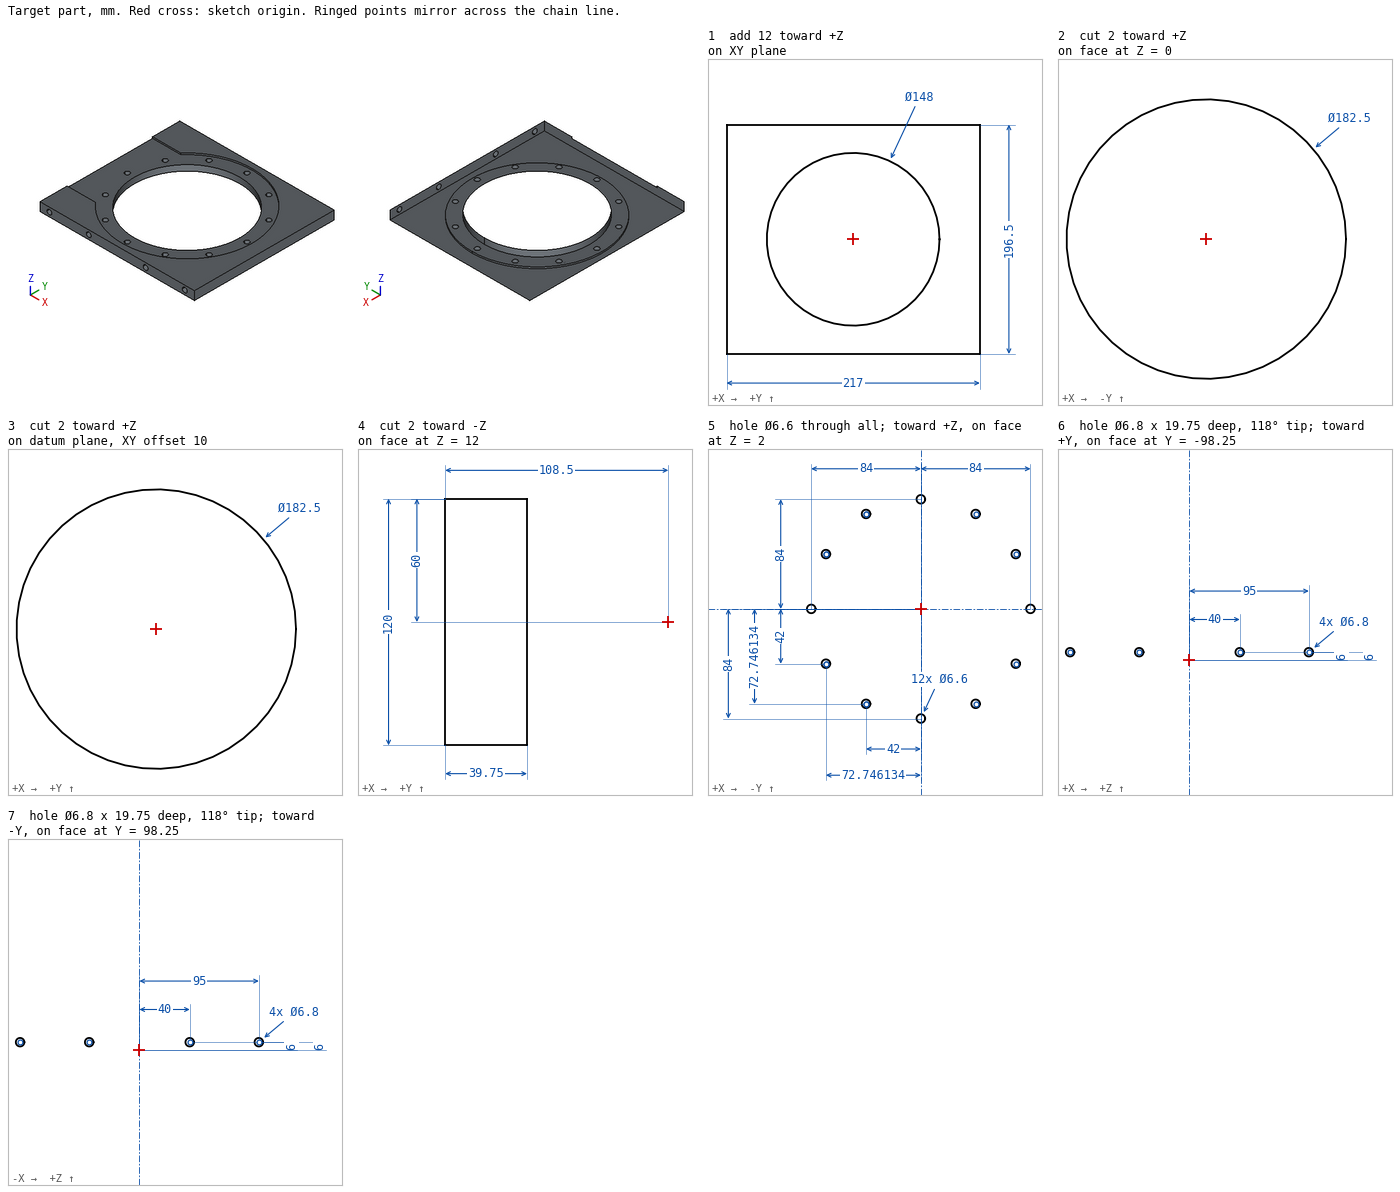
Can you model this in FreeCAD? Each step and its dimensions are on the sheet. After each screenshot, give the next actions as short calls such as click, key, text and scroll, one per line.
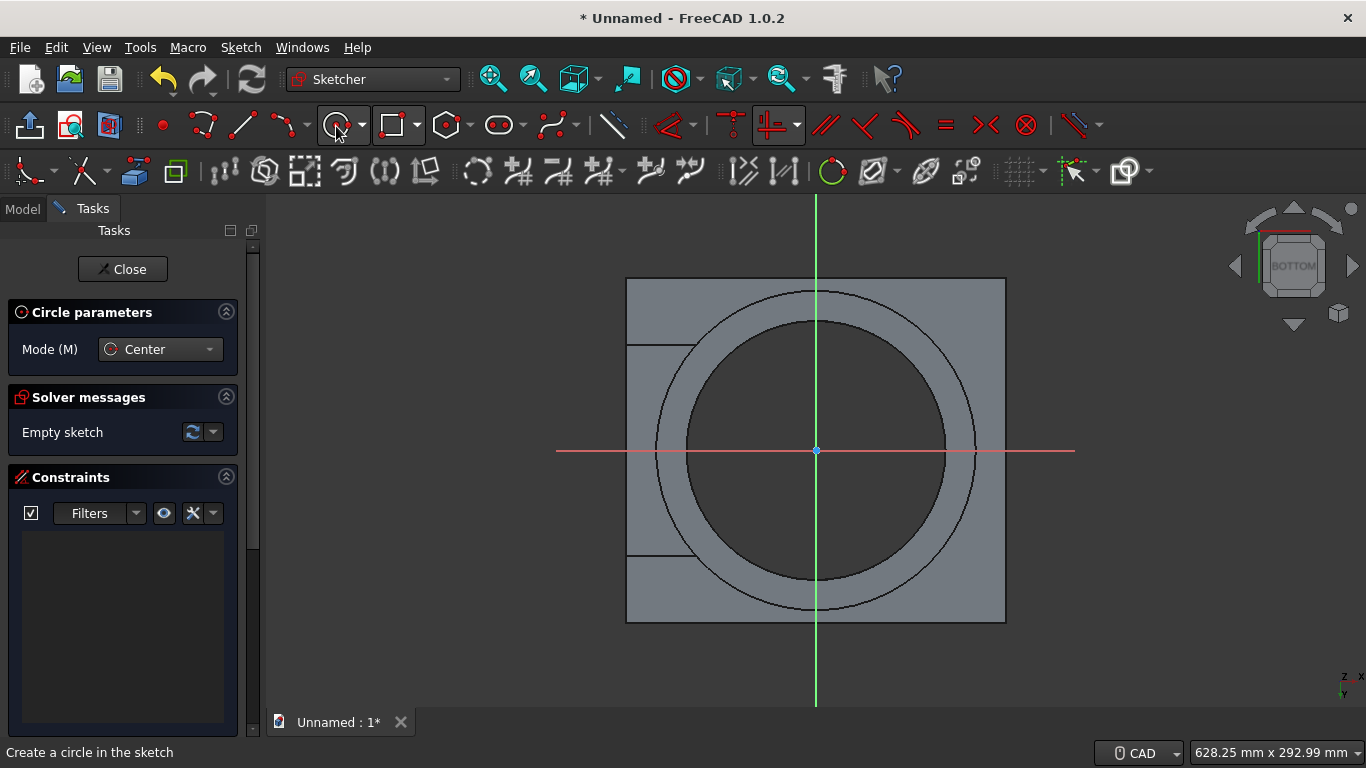
scroll(816, 598, up, 7)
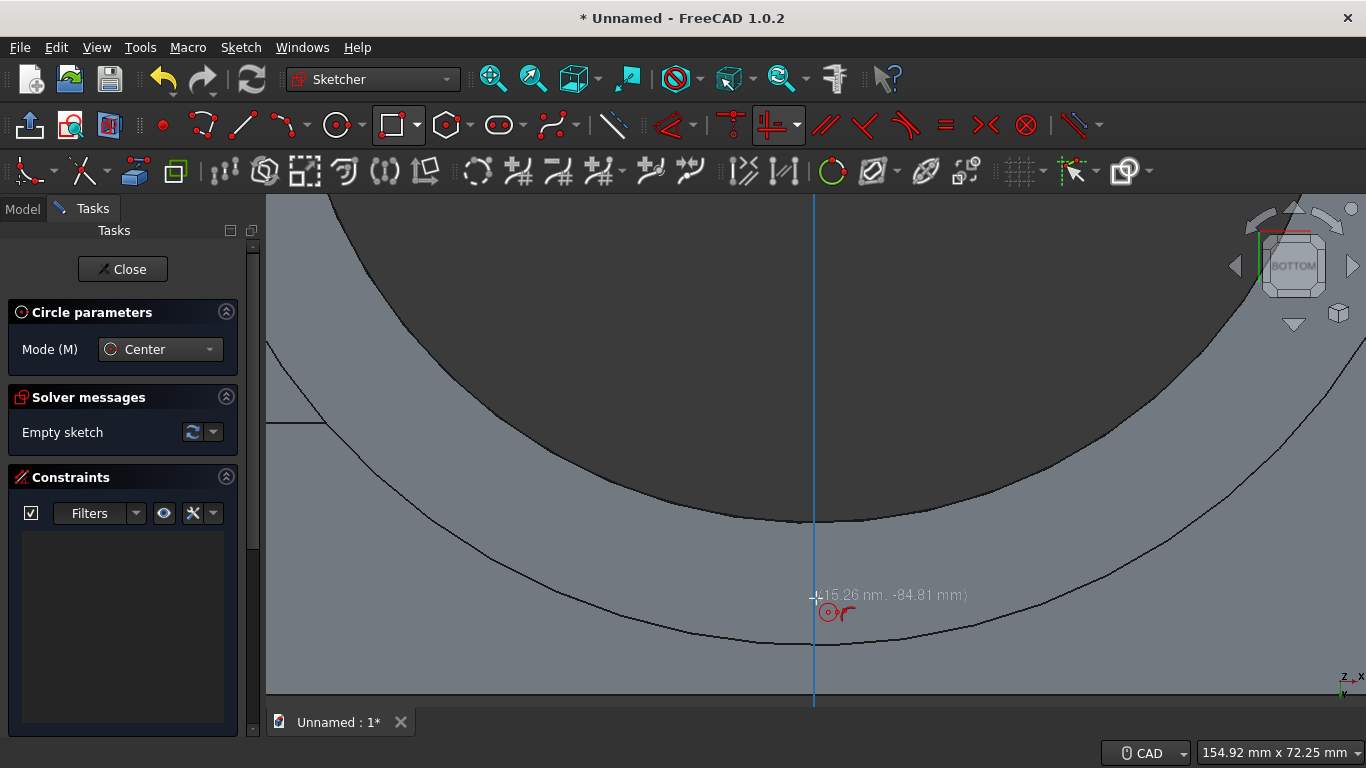
scroll(726, 599, down, 7)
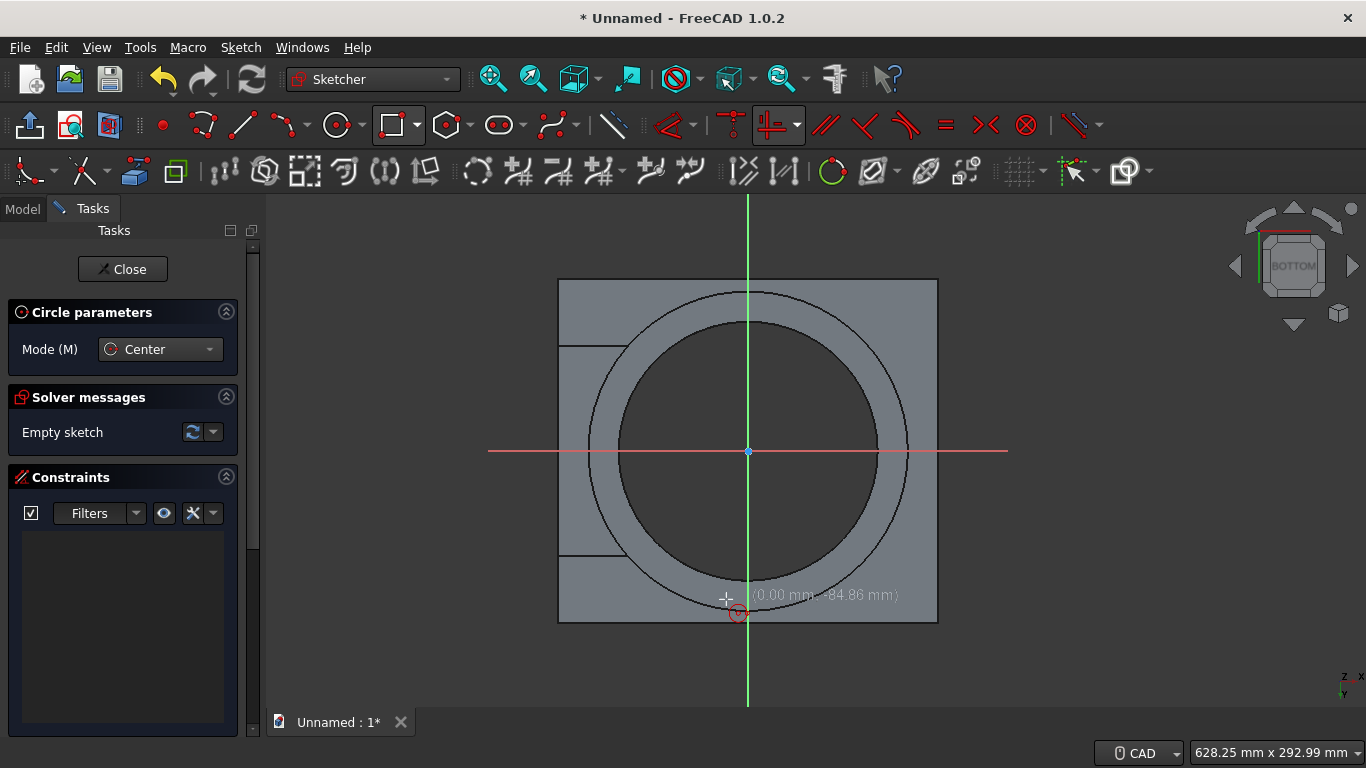
click(748, 598)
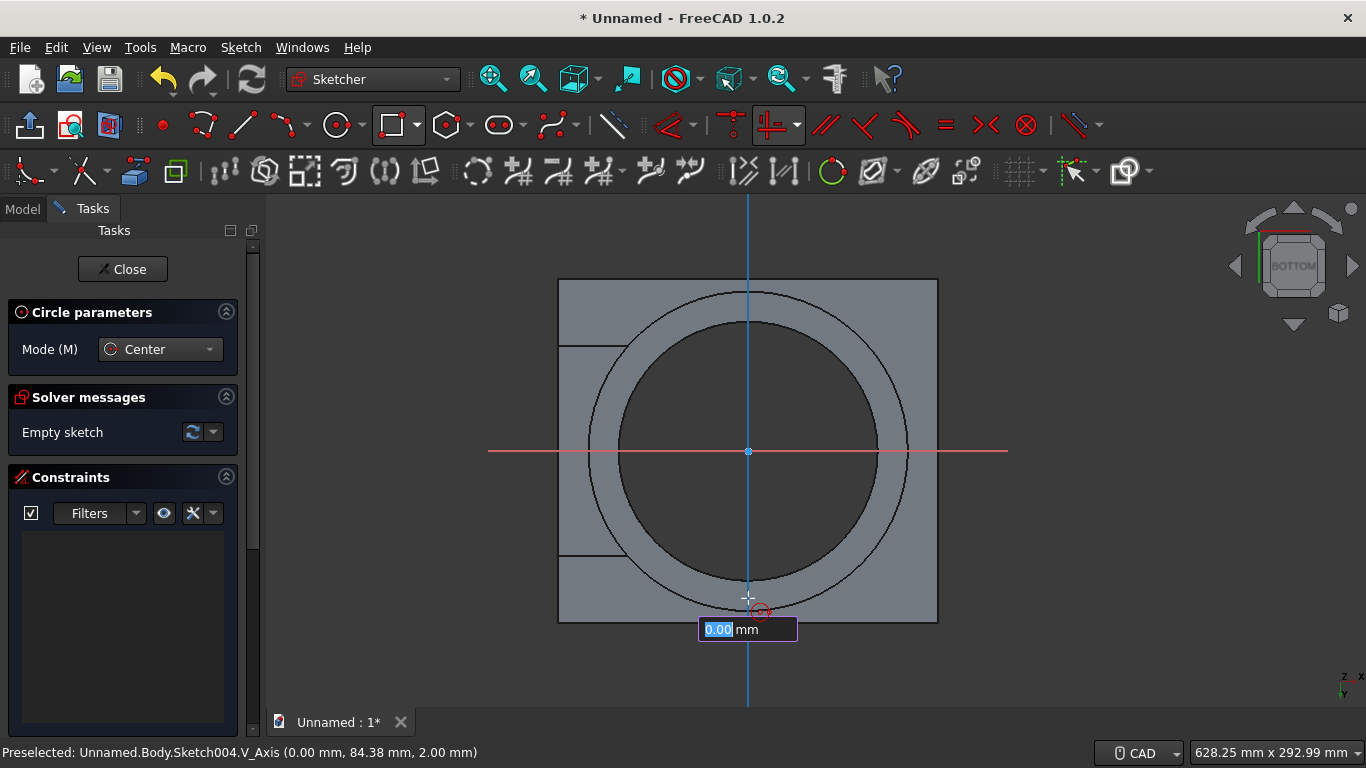
scroll(754, 596, up, 6)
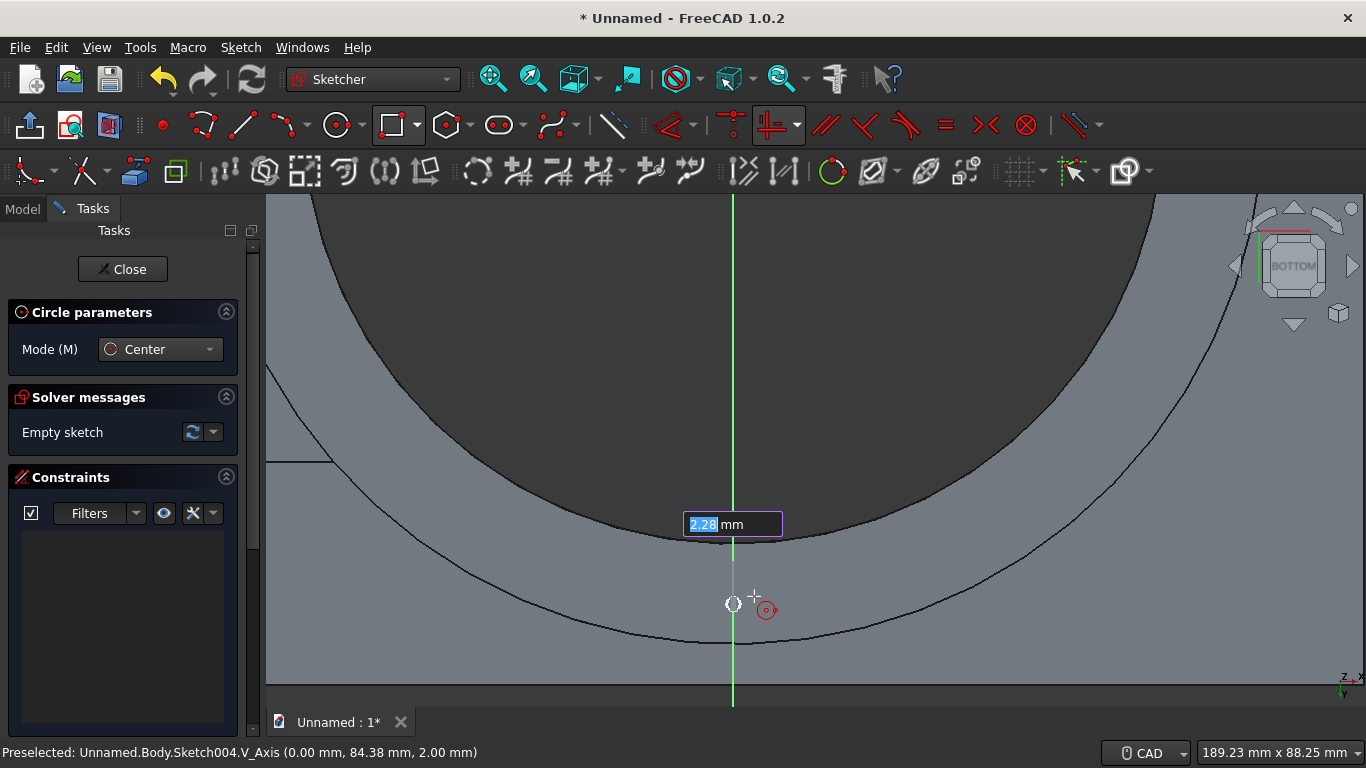
click(752, 595)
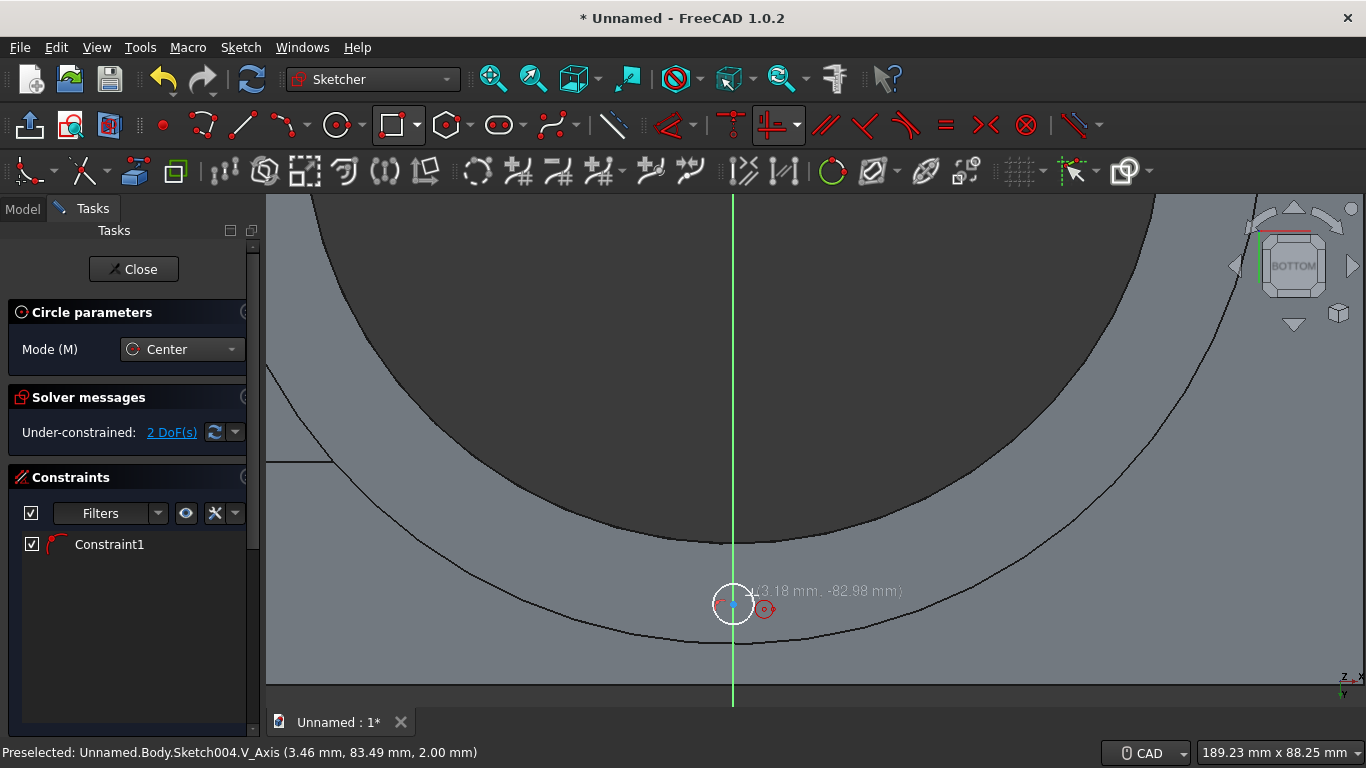
click(489, 536)
click(503, 523)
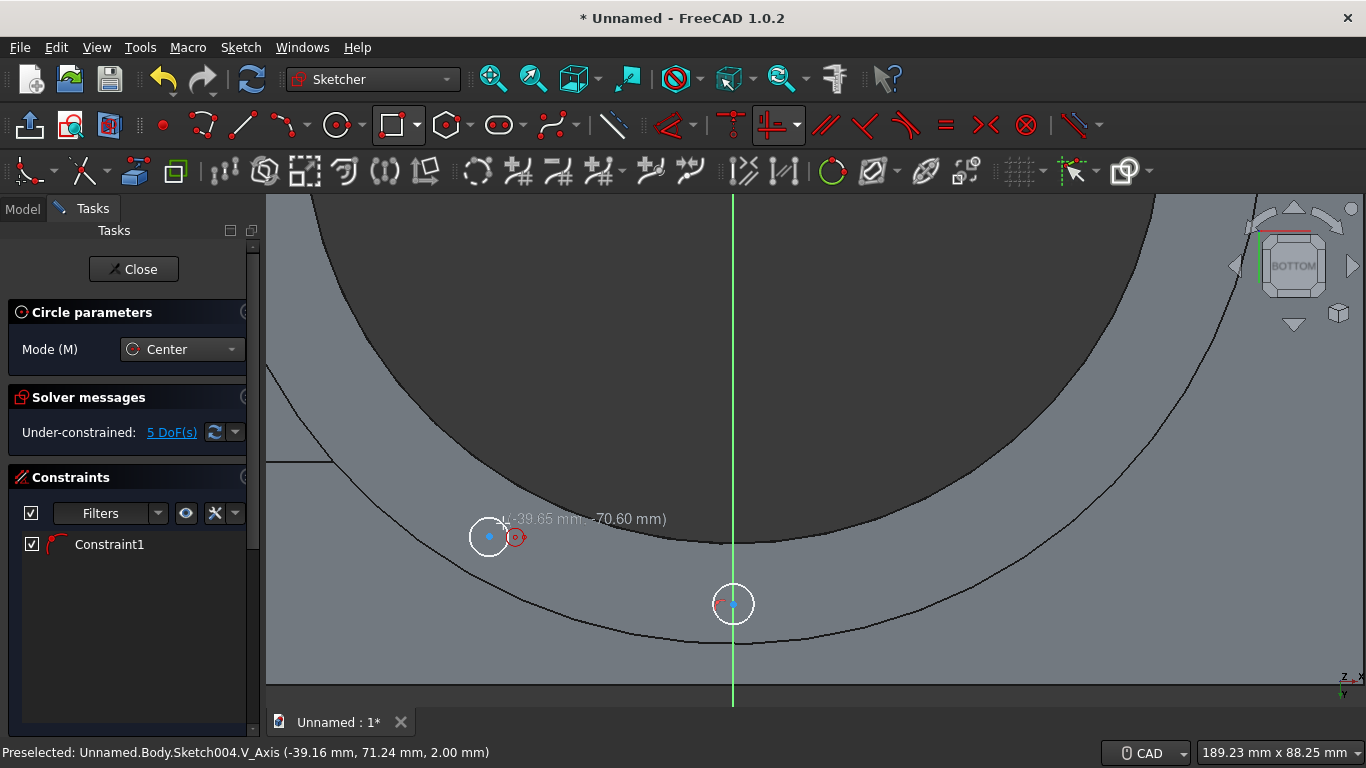
click(311, 358)
click(324, 344)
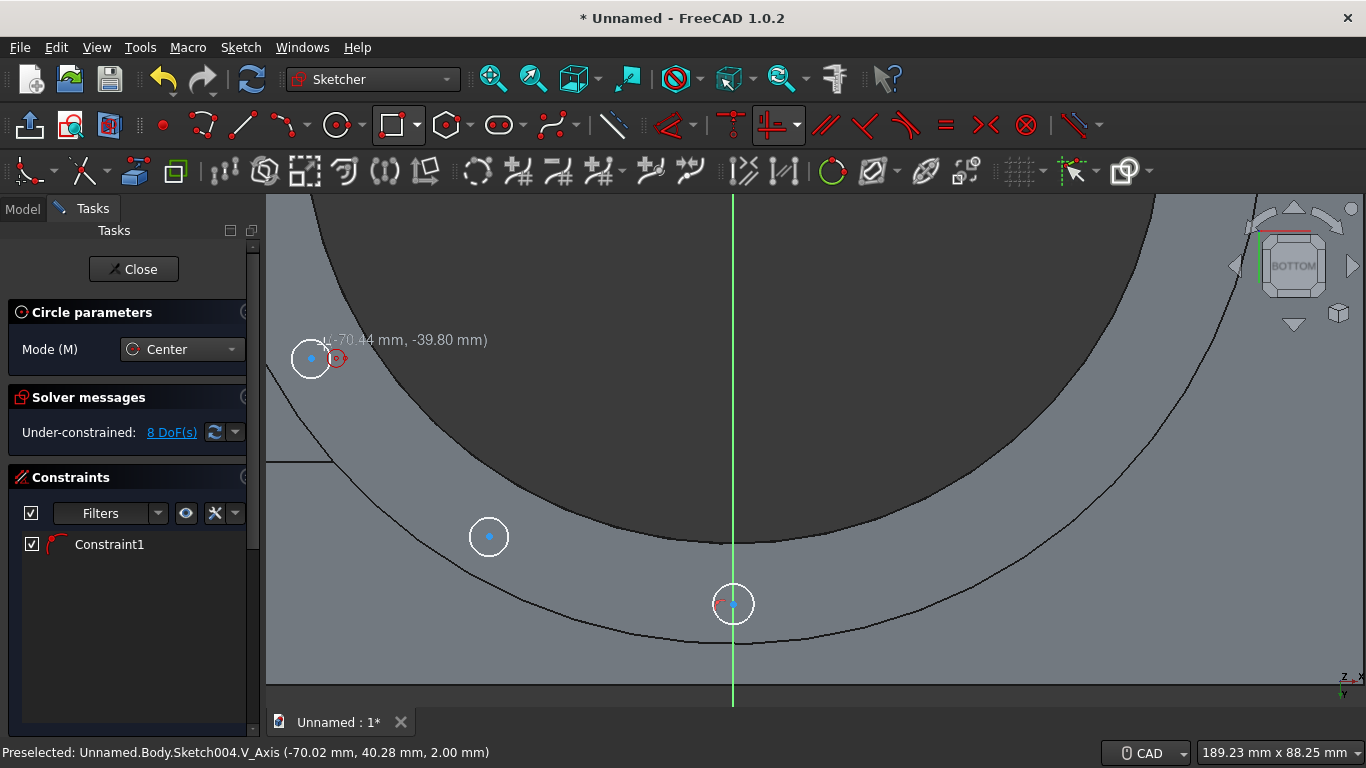
scroll(754, 596, down, 6)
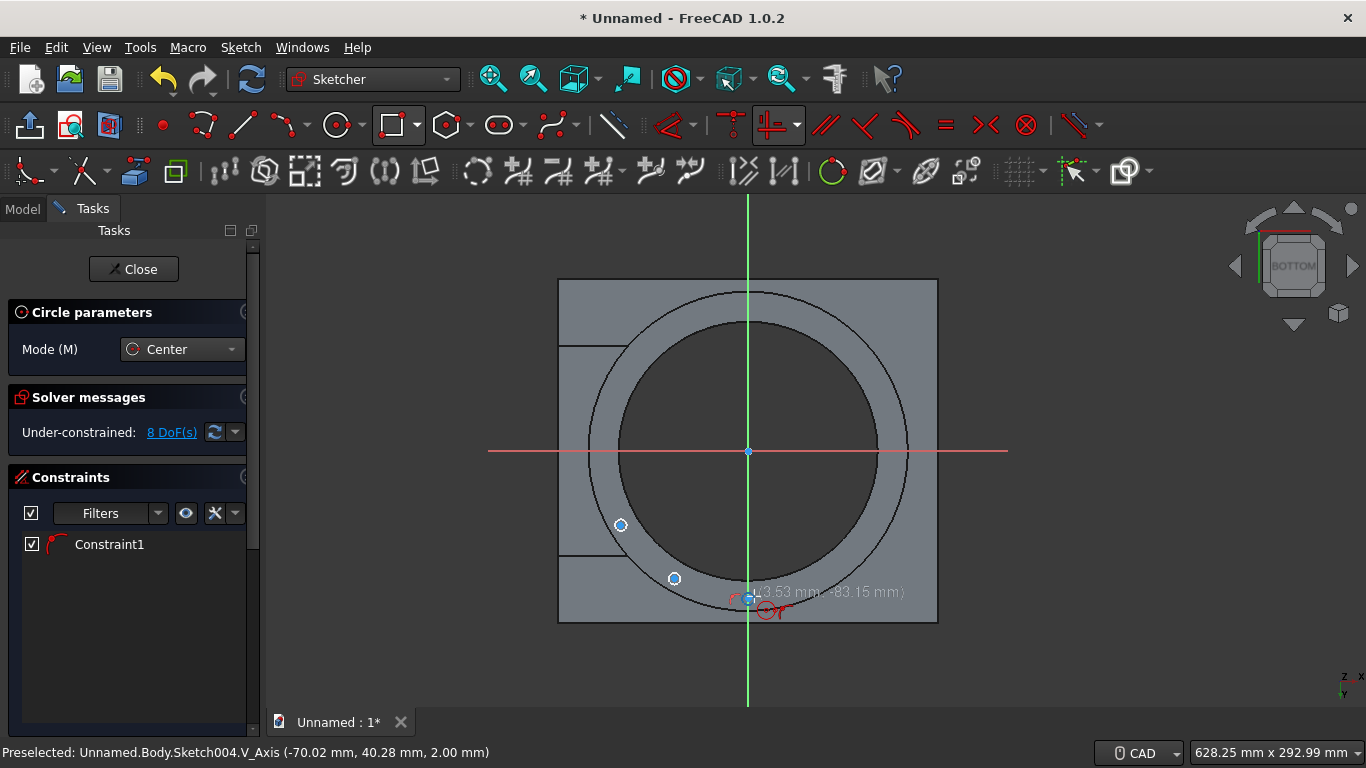
scroll(601, 451, up, 7)